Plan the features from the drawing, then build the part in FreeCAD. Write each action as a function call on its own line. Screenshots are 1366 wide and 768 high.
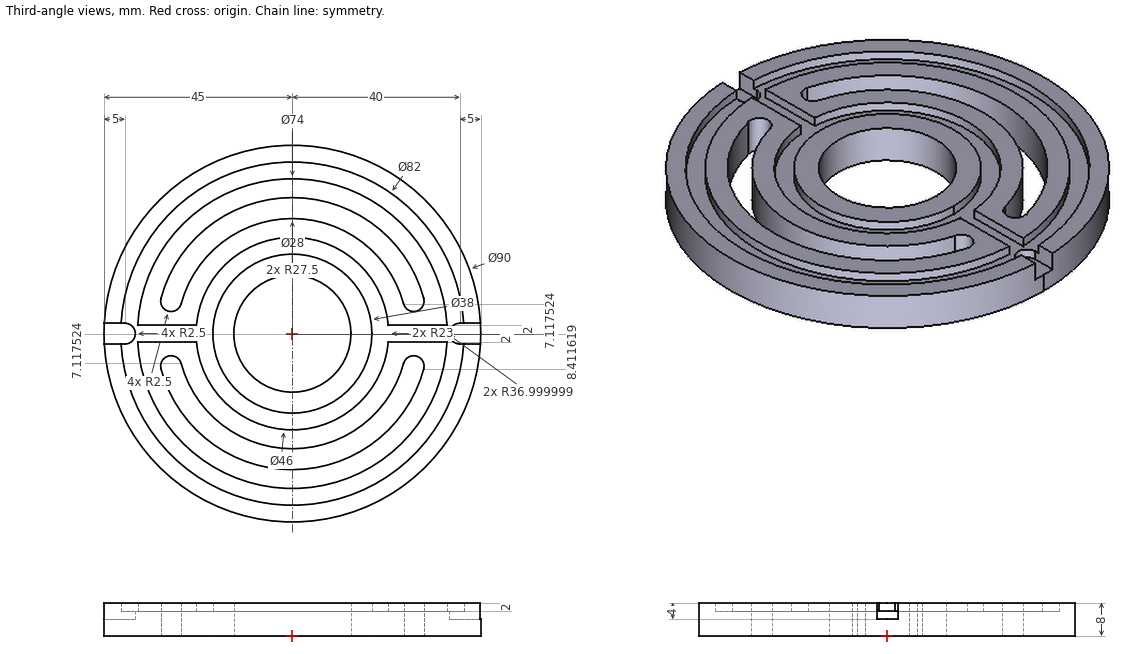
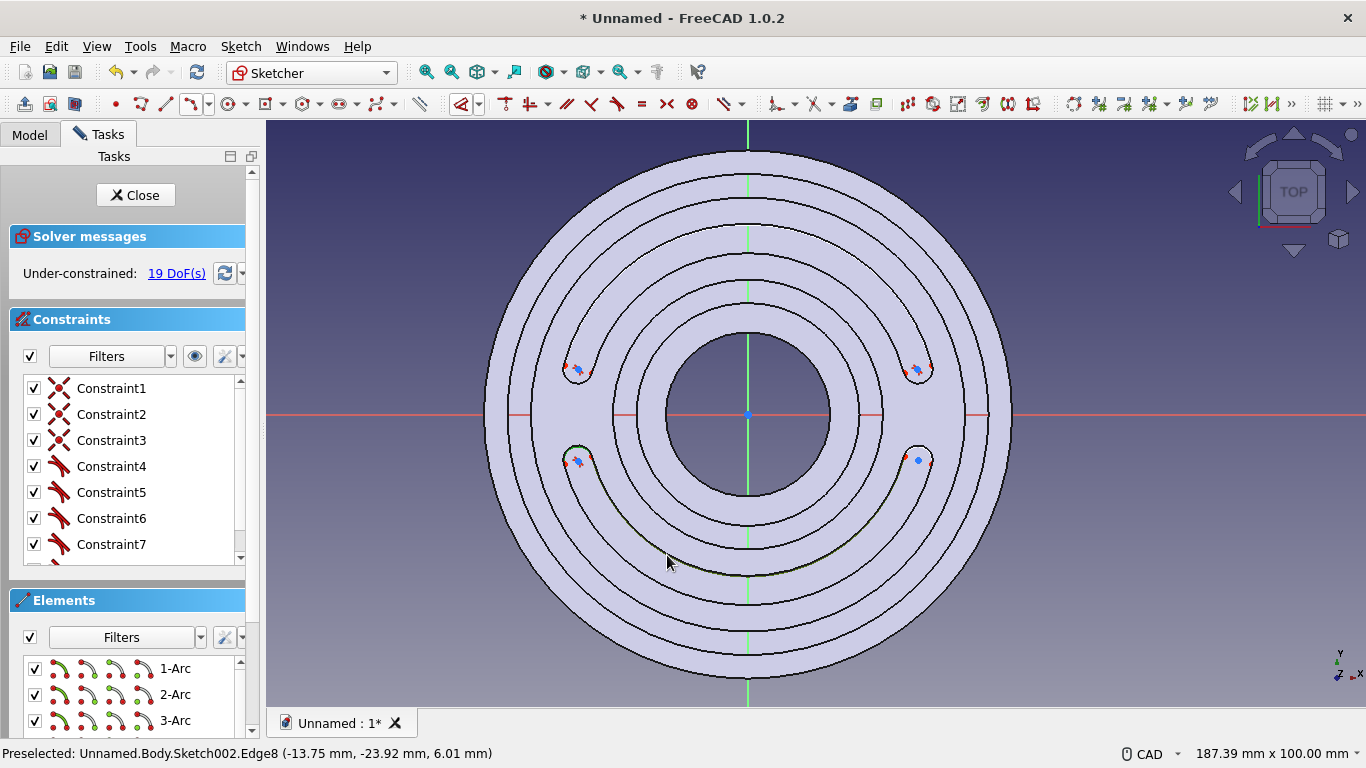
click(617, 104)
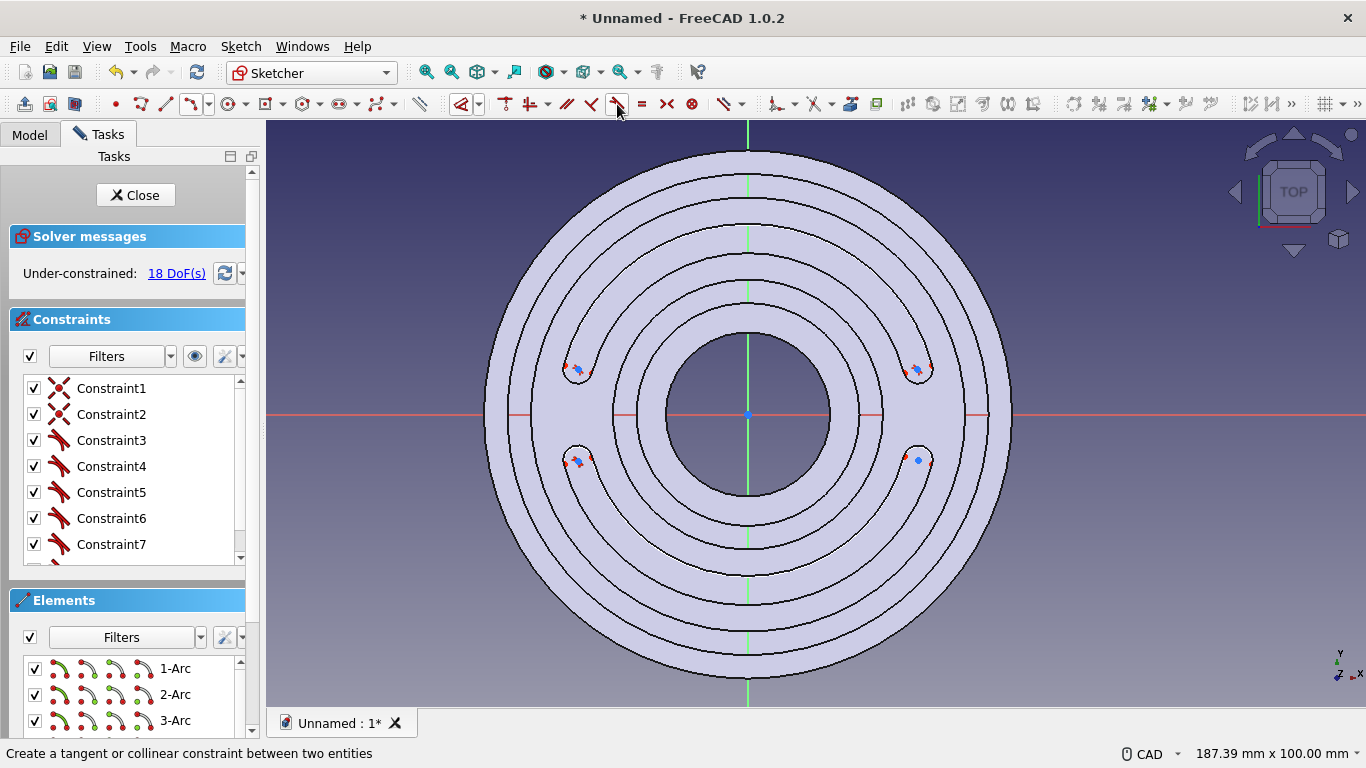
click(653, 581)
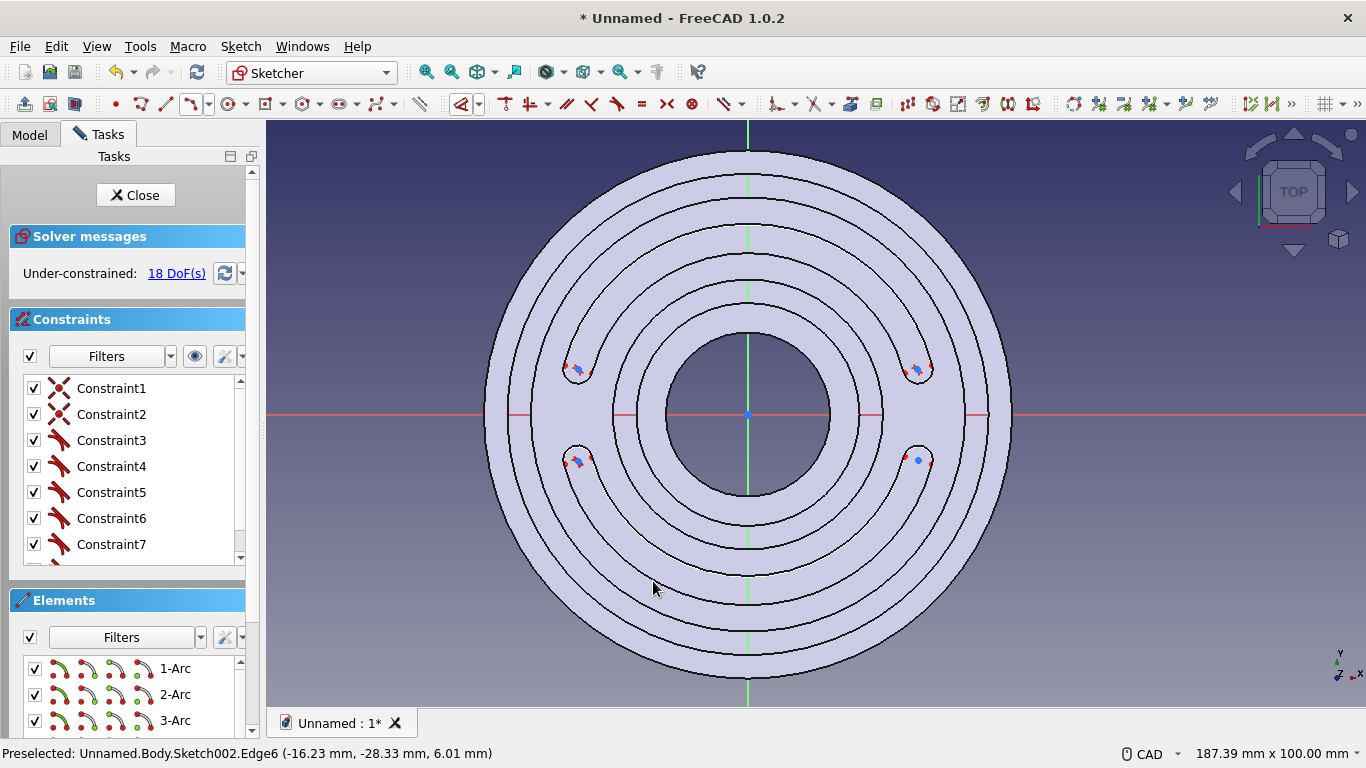
click(929, 452)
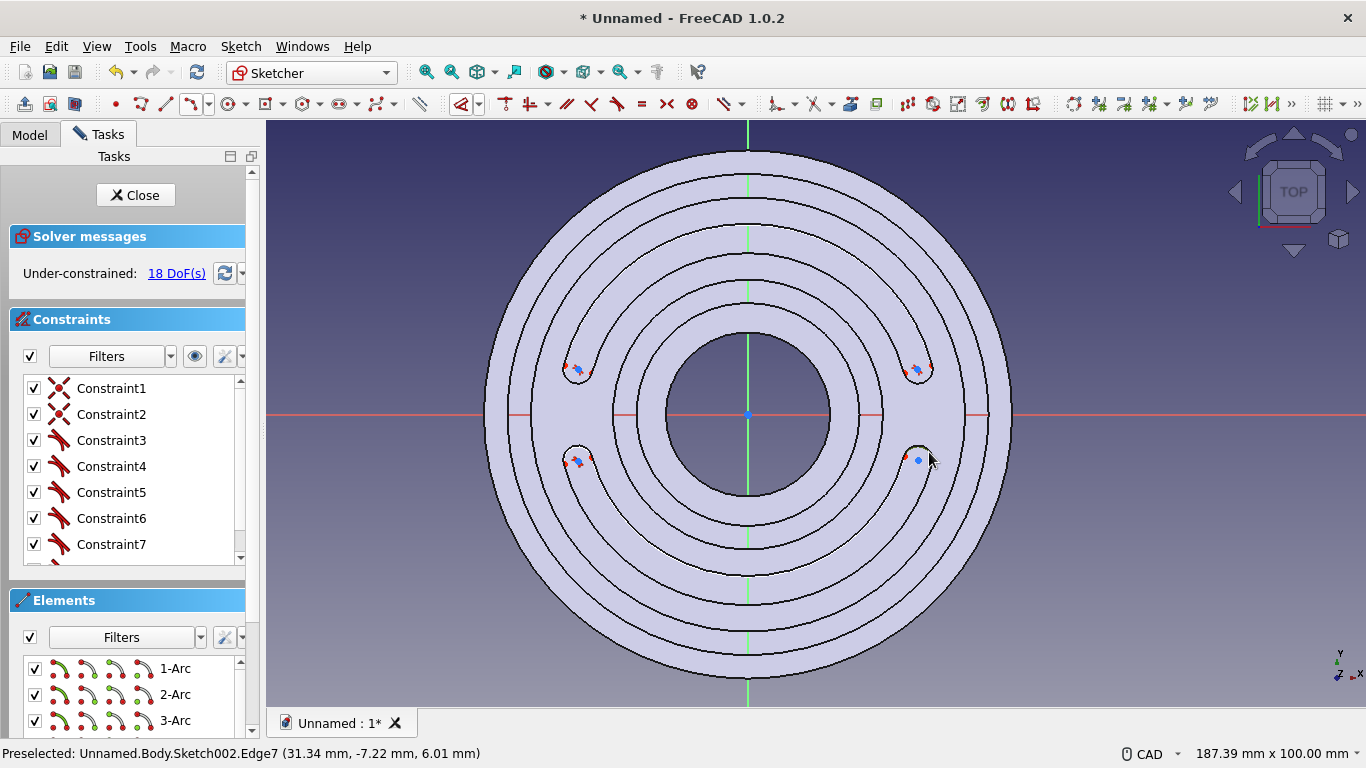
key(t)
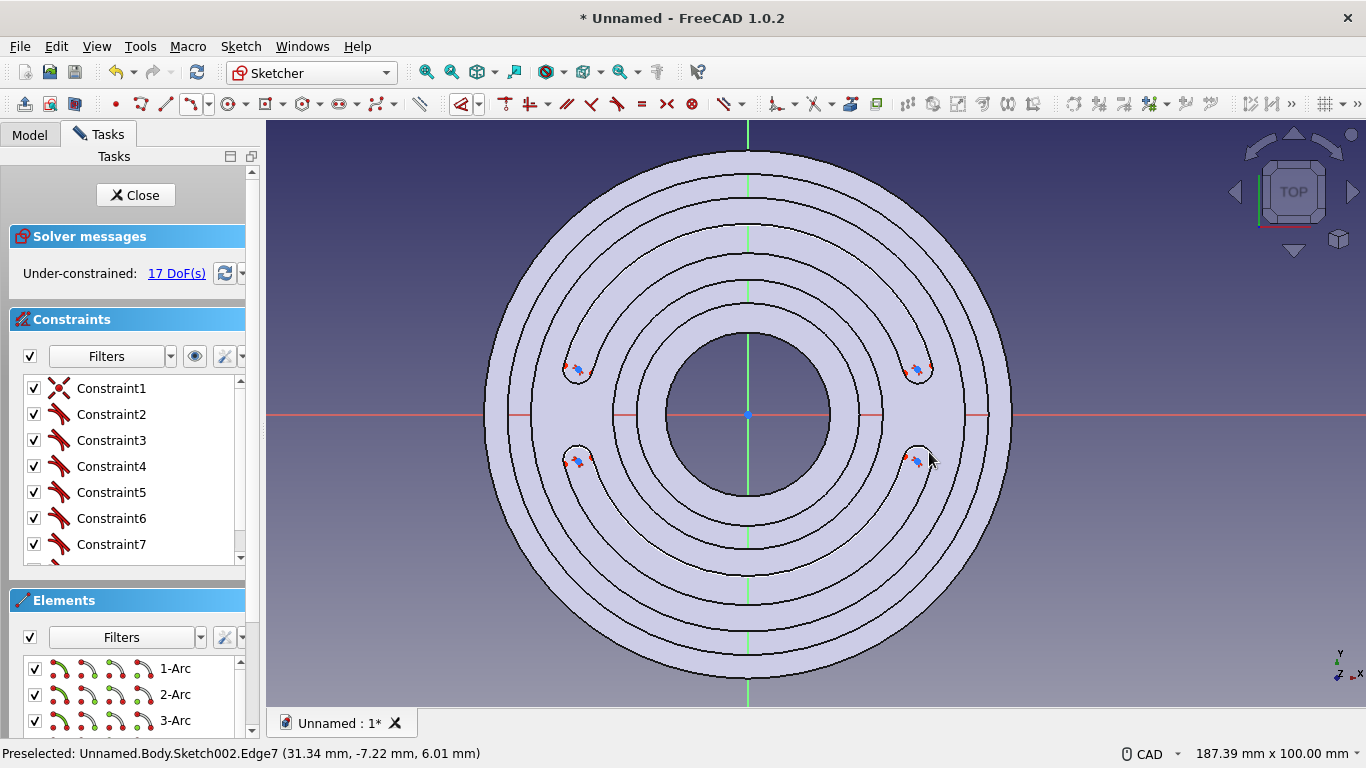
click(929, 452)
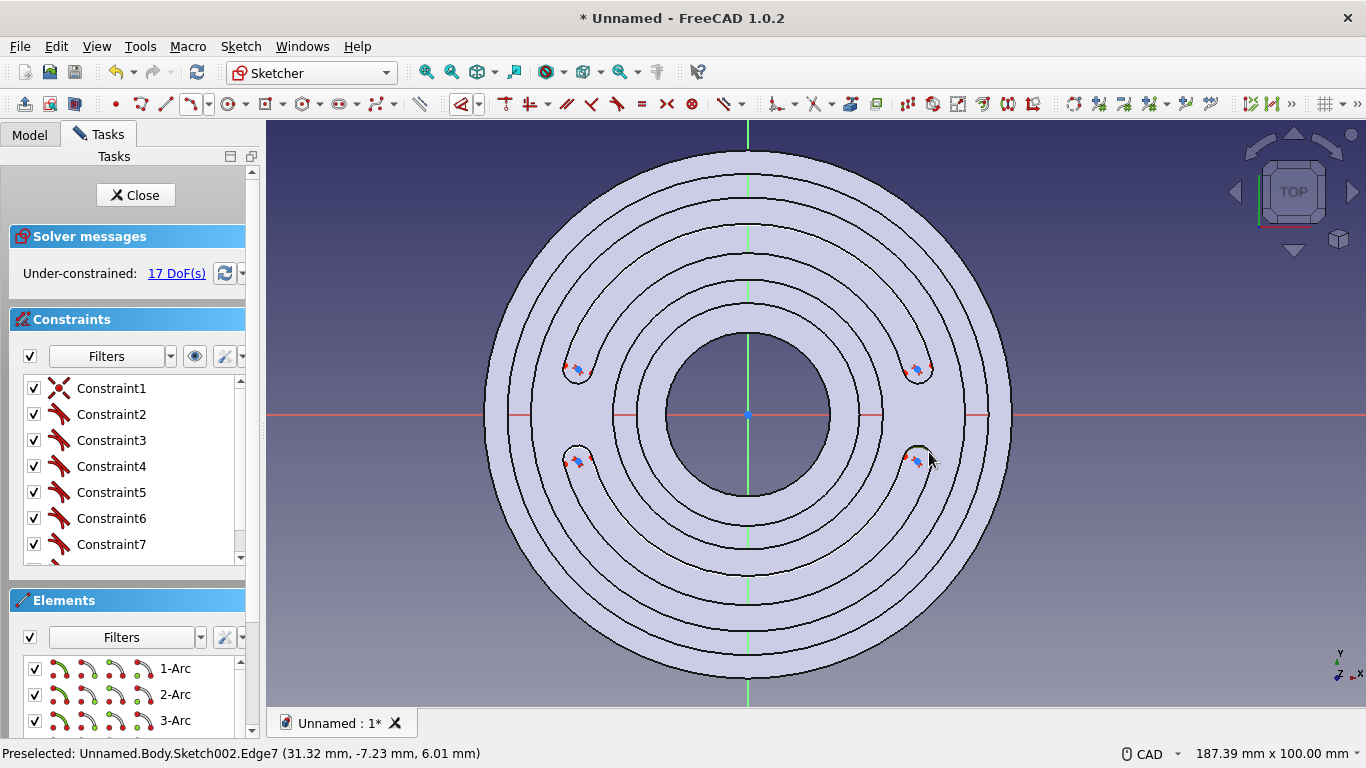
click(667, 555)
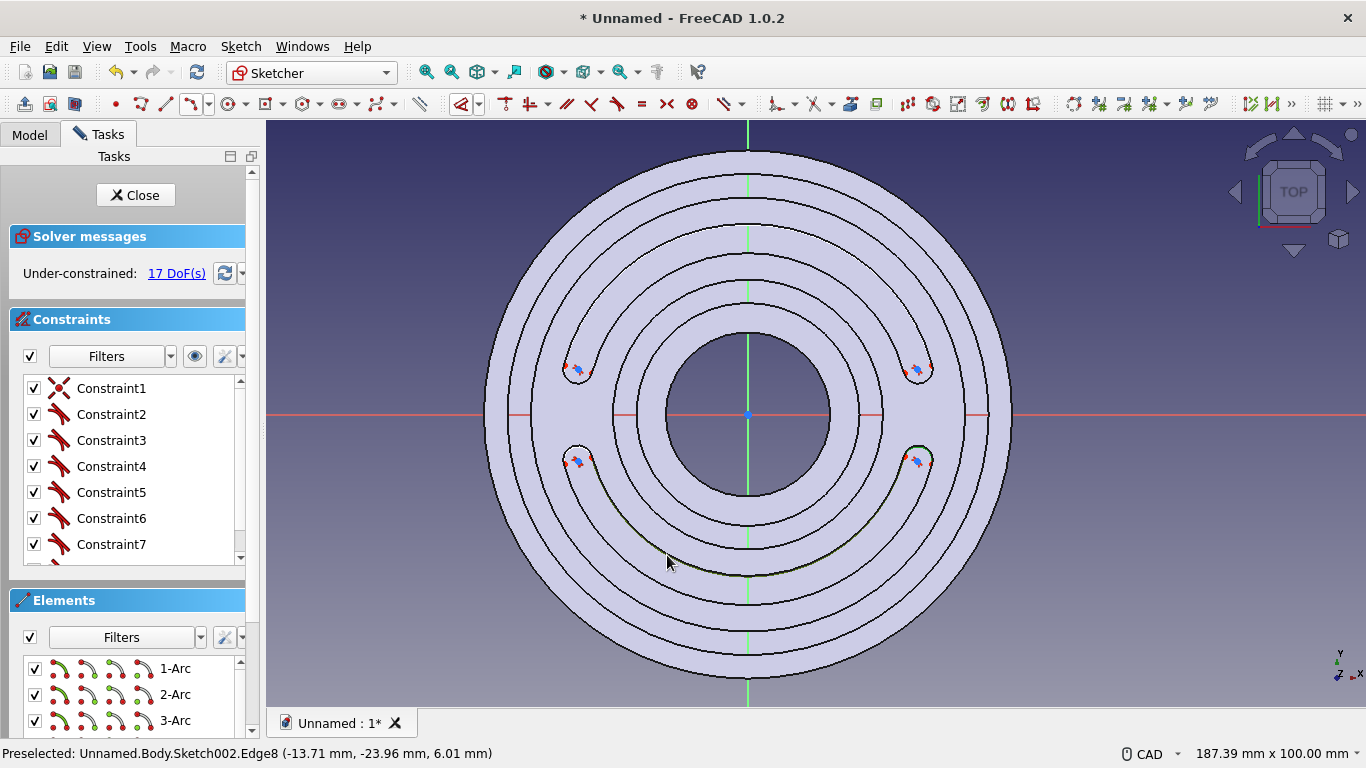
key(t)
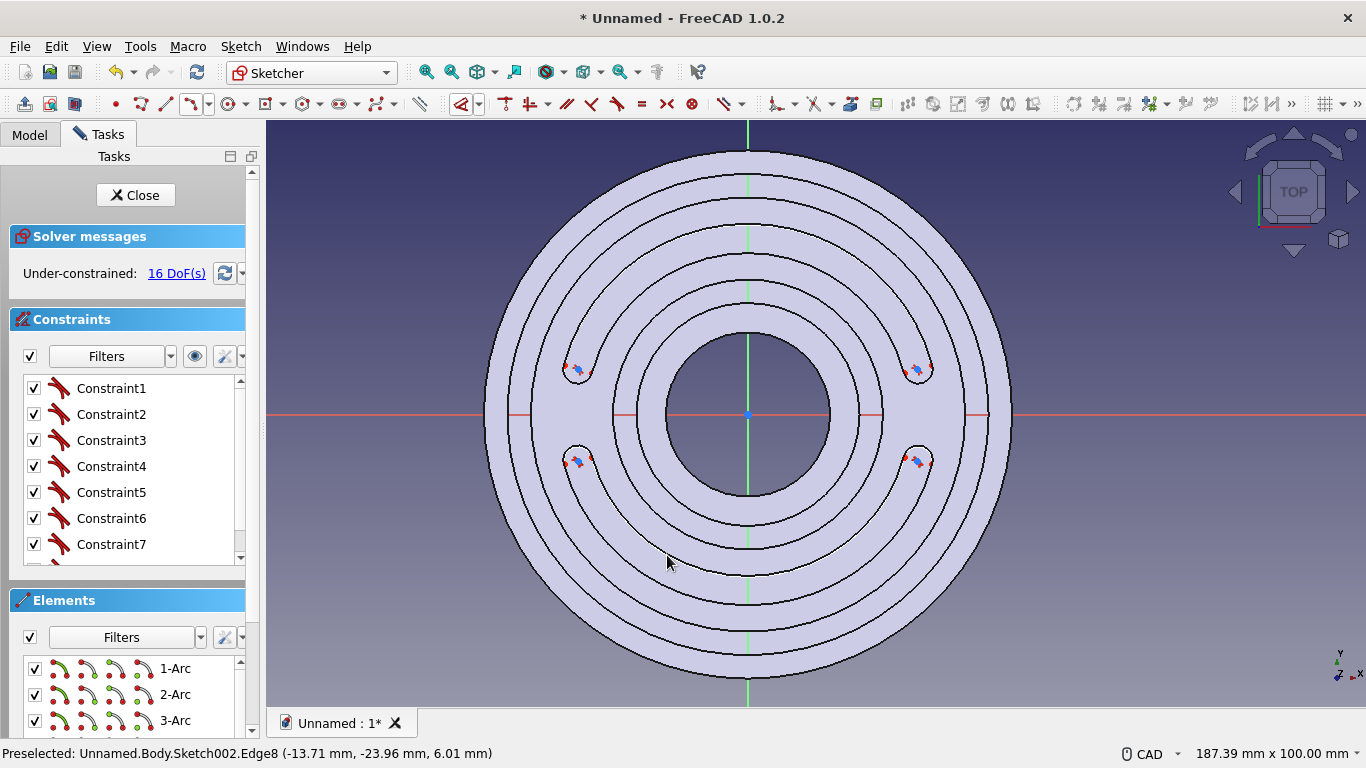
click(829, 276)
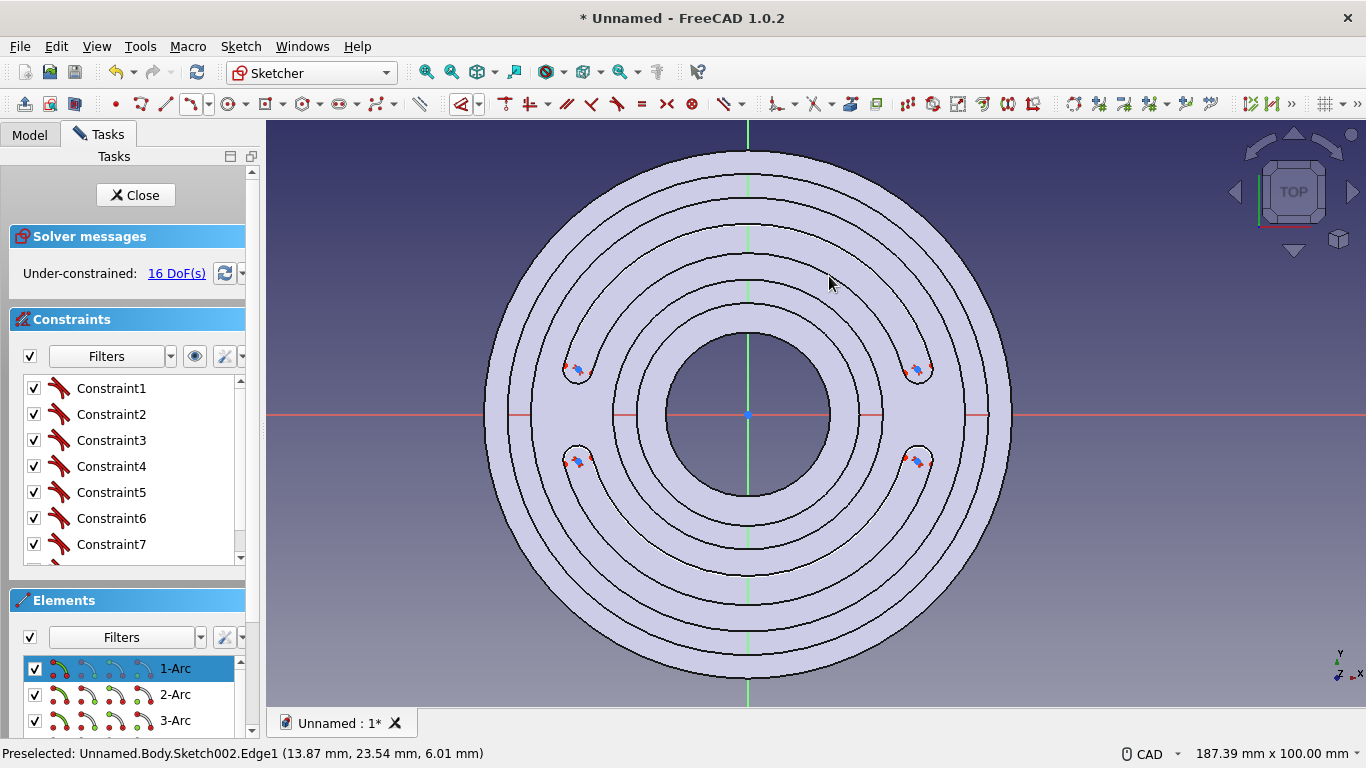
click(843, 250)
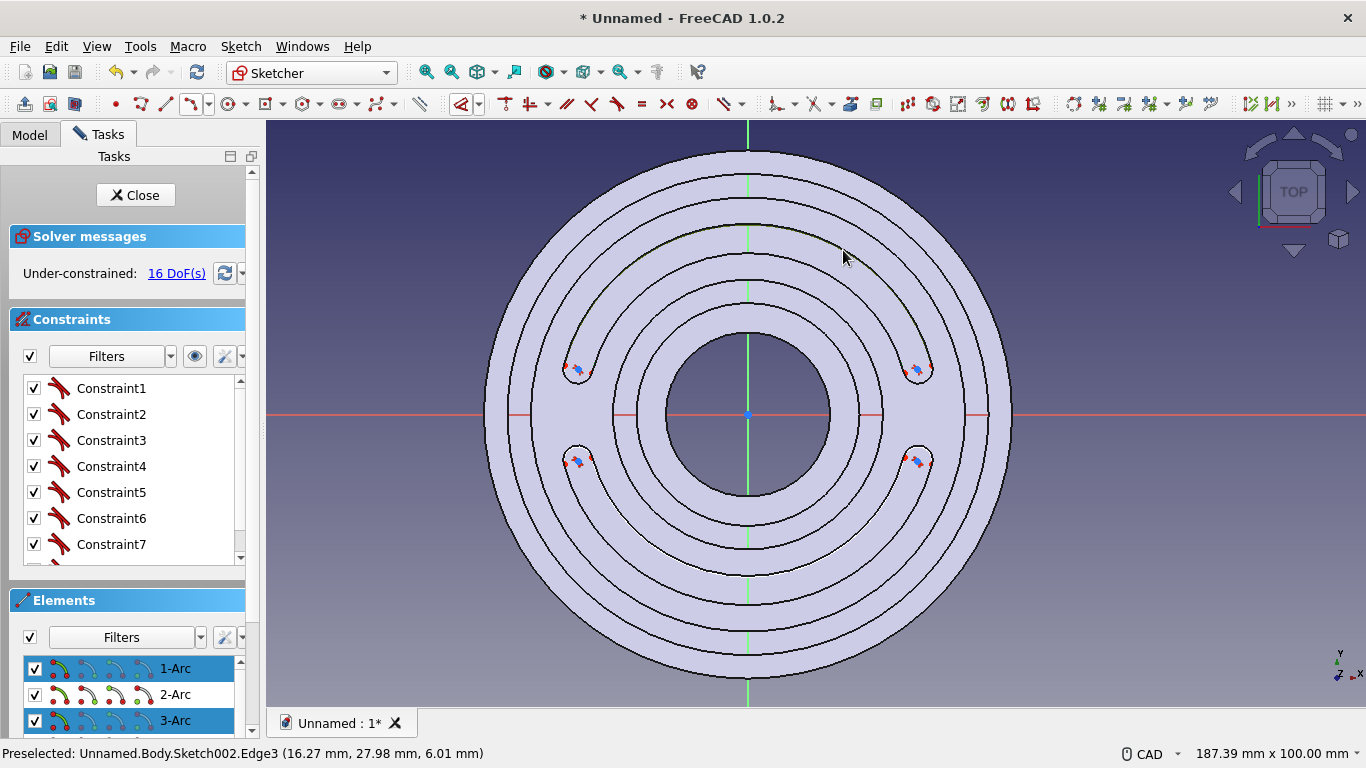
key(c)